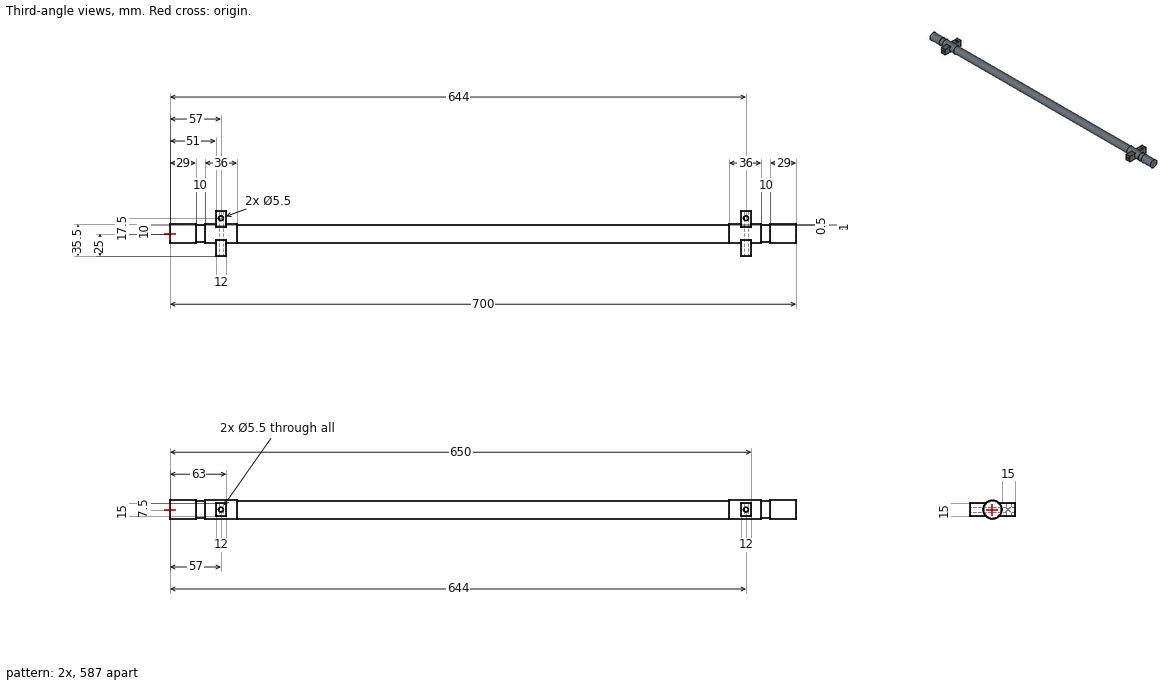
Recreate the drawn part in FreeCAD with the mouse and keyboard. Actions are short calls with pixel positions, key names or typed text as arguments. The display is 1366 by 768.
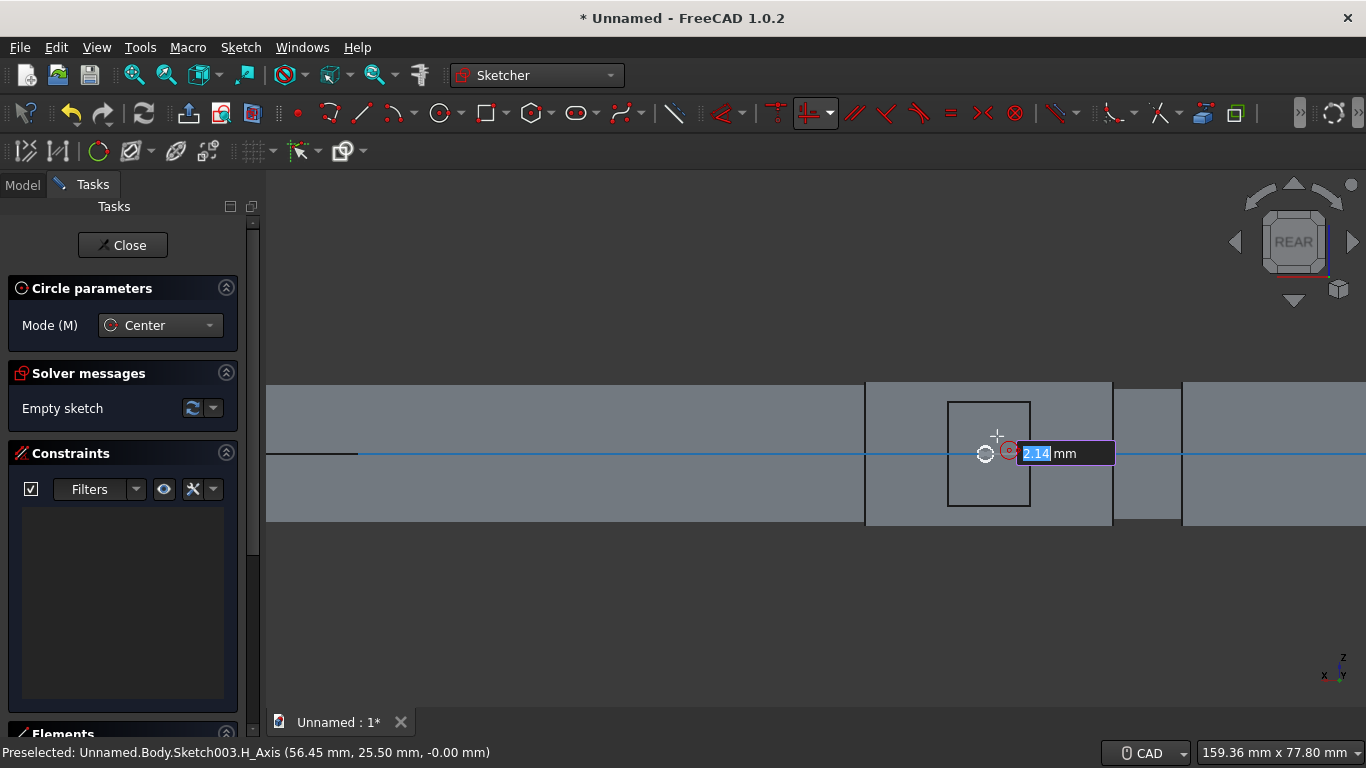
click(995, 436)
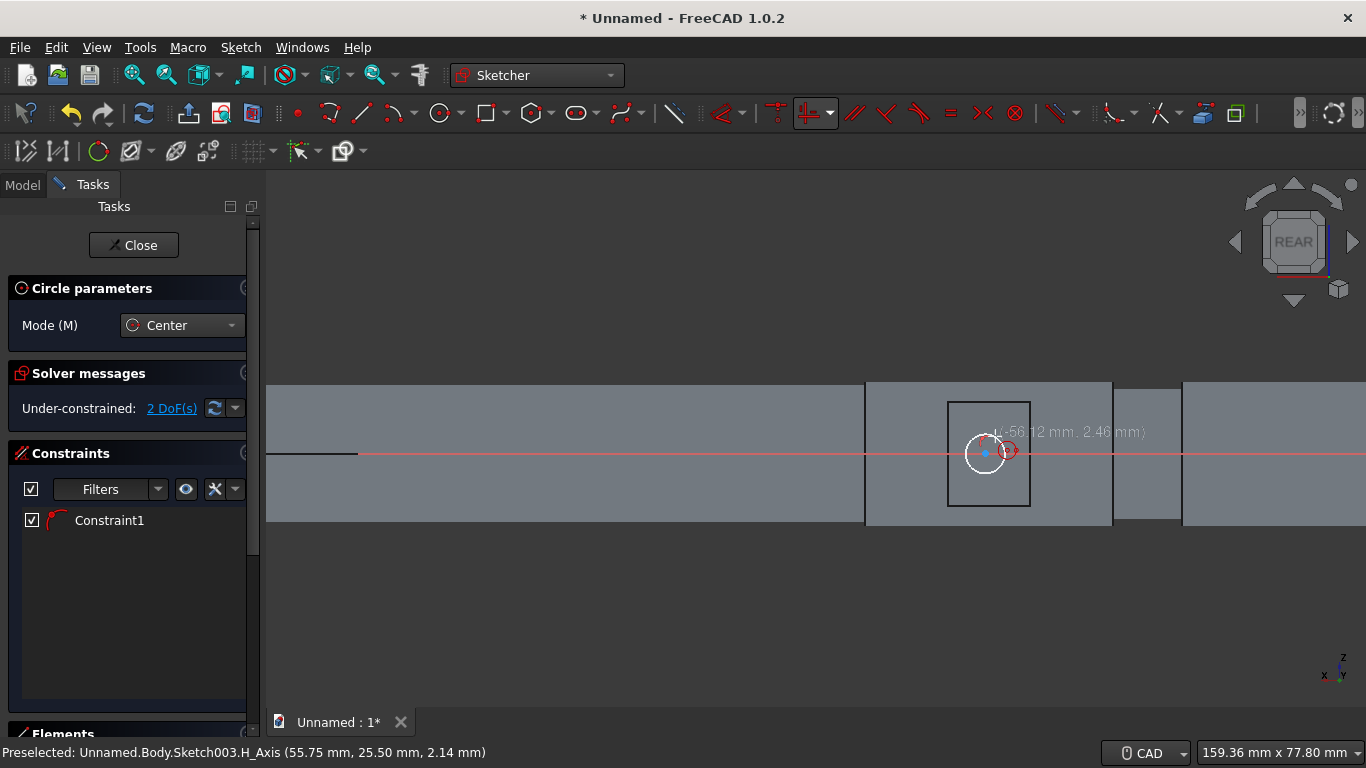
scroll(997, 436, down, 10)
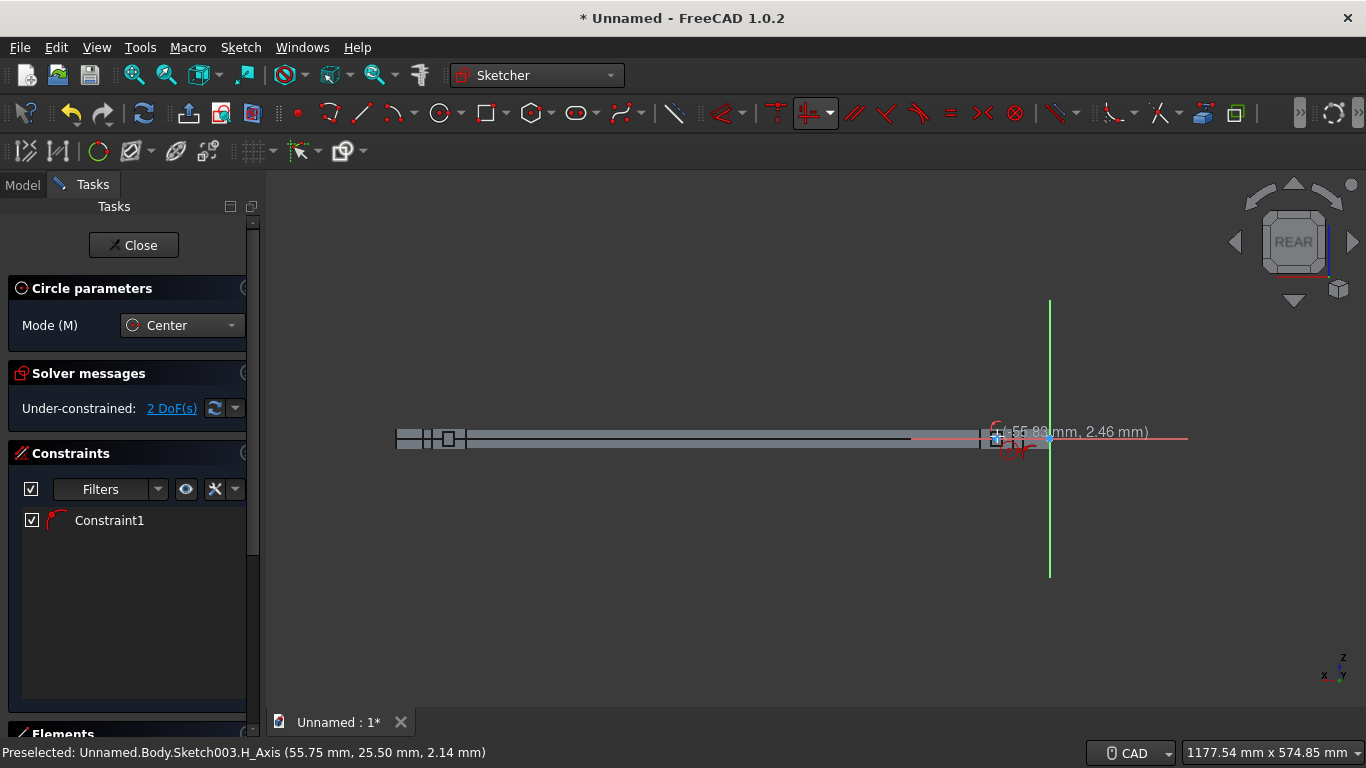
scroll(448, 439, up, 11)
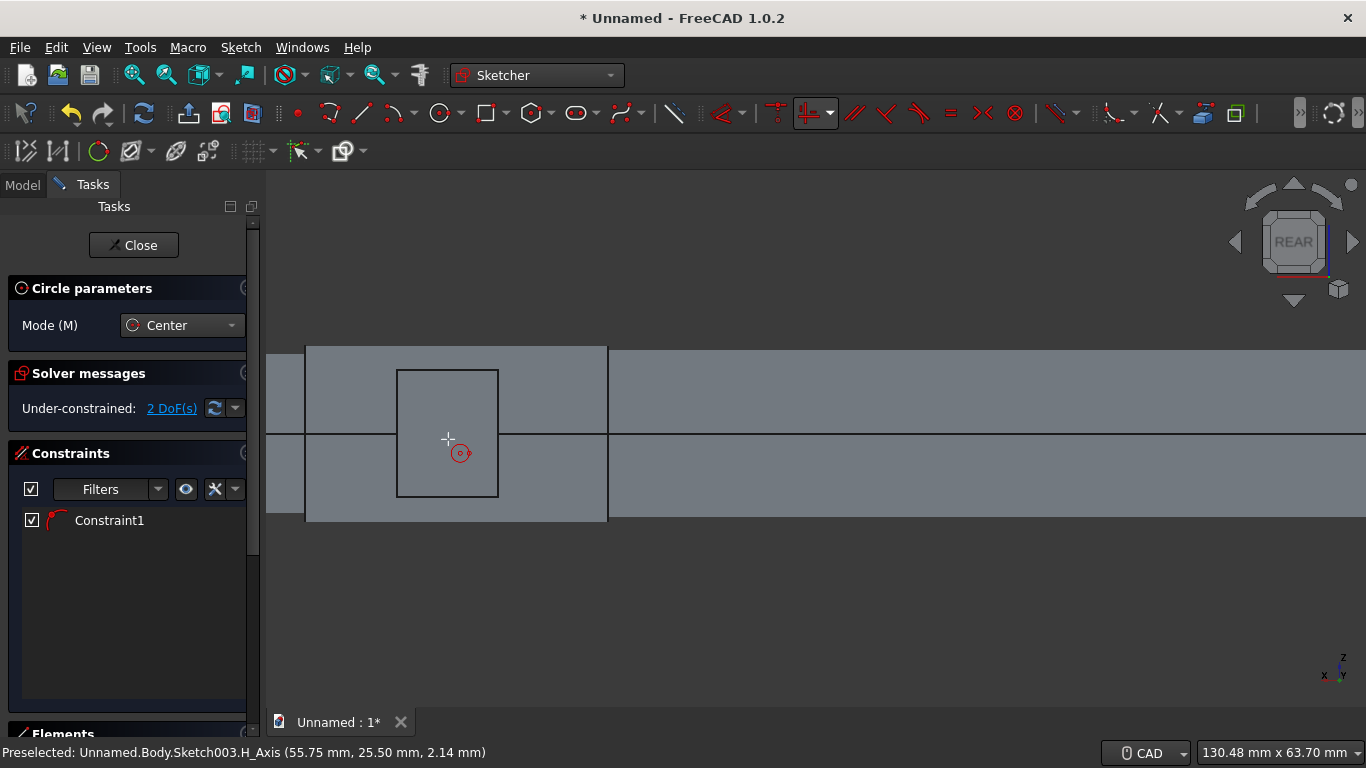
scroll(448, 439, down, 11)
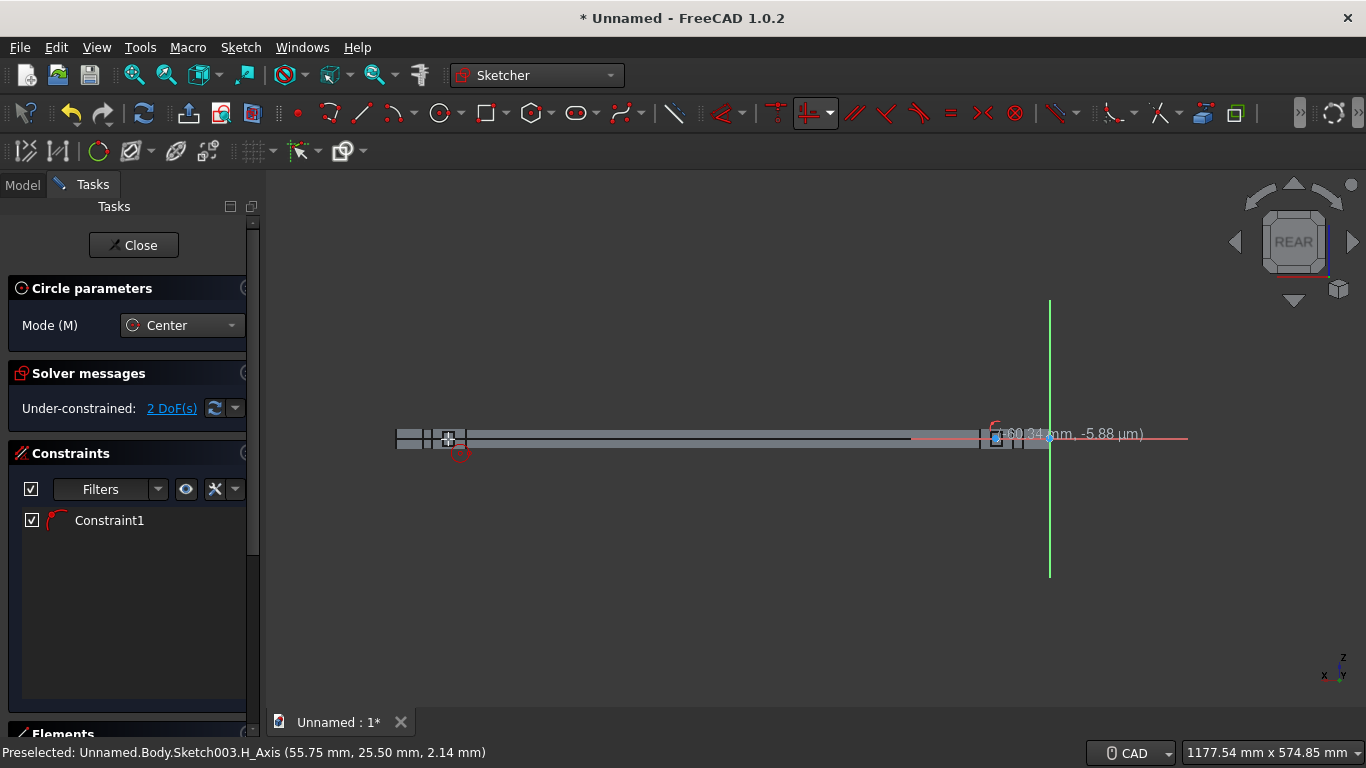
click(448, 439)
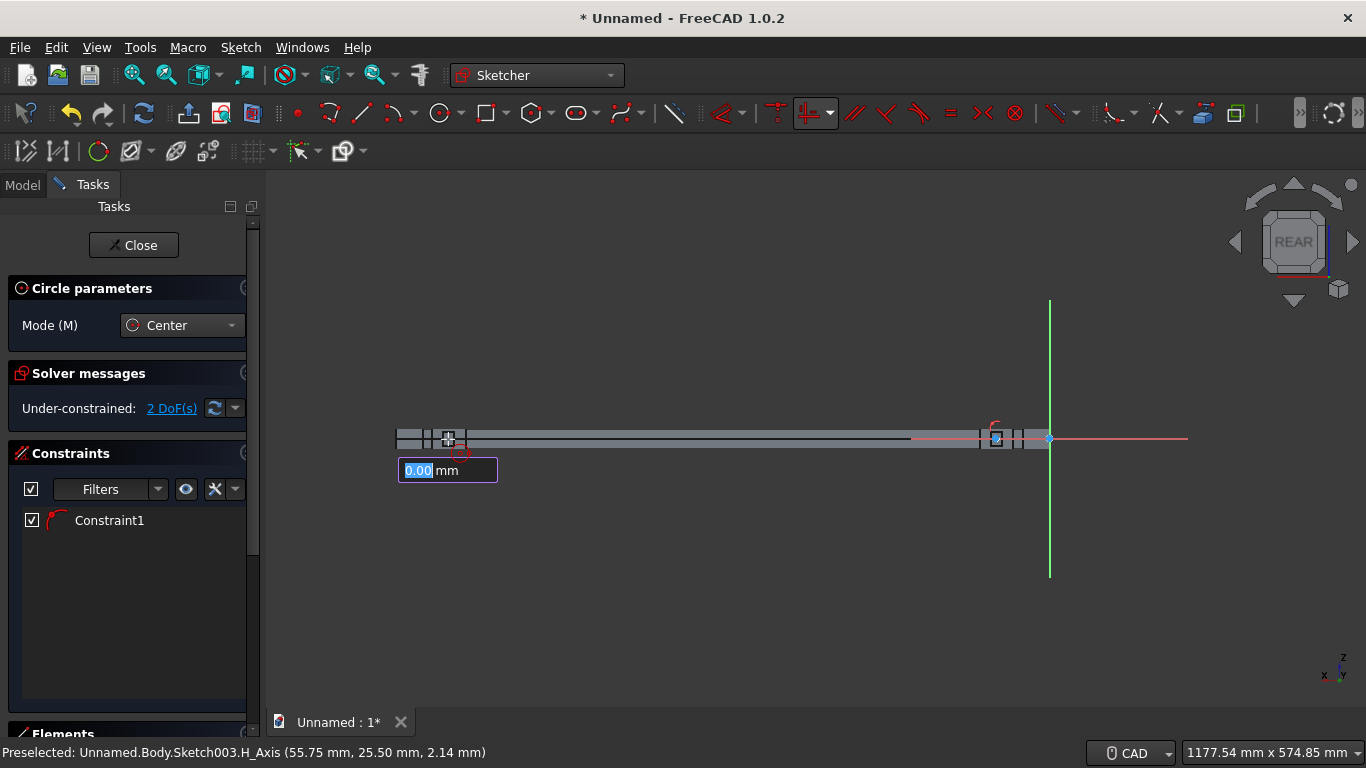
scroll(449, 436, up, 10)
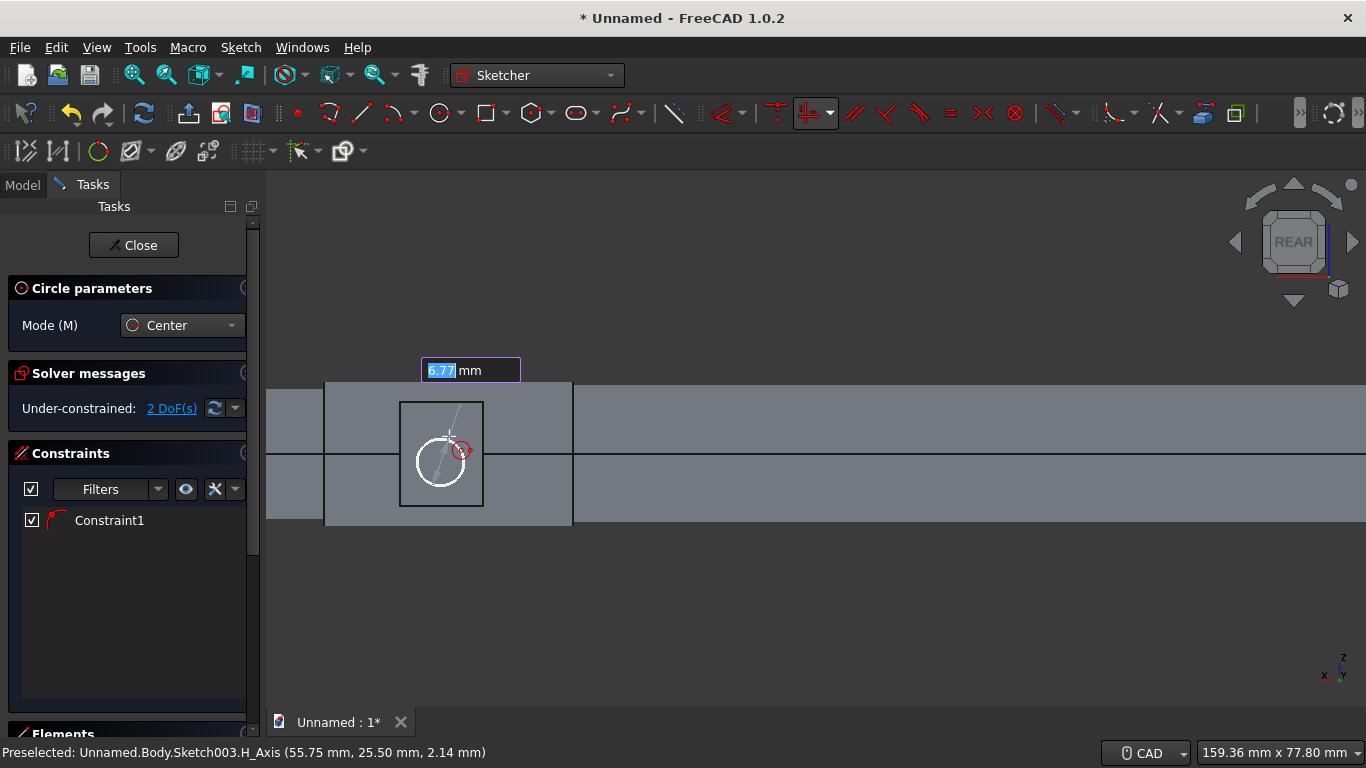
click(448, 436)
key(Escape)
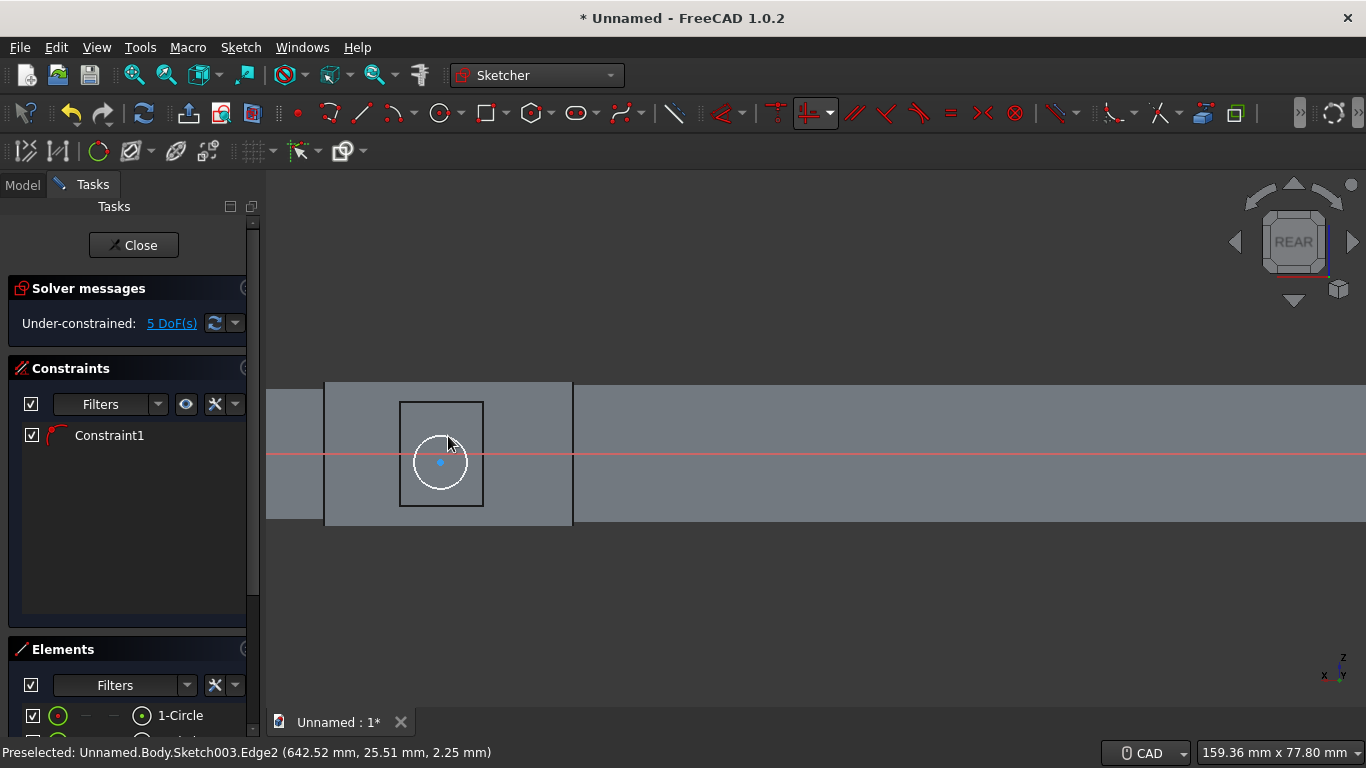
scroll(449, 436, down, 10)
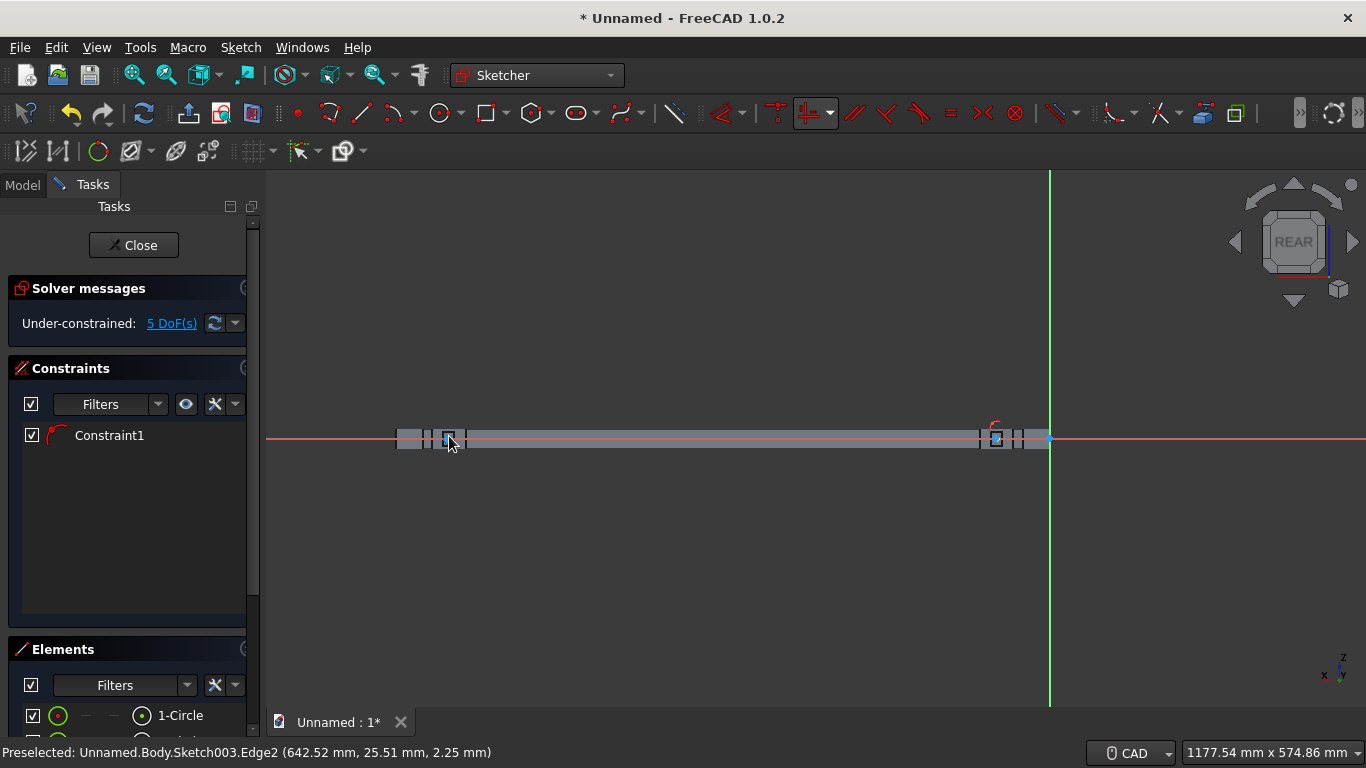
scroll(998, 437, up, 10)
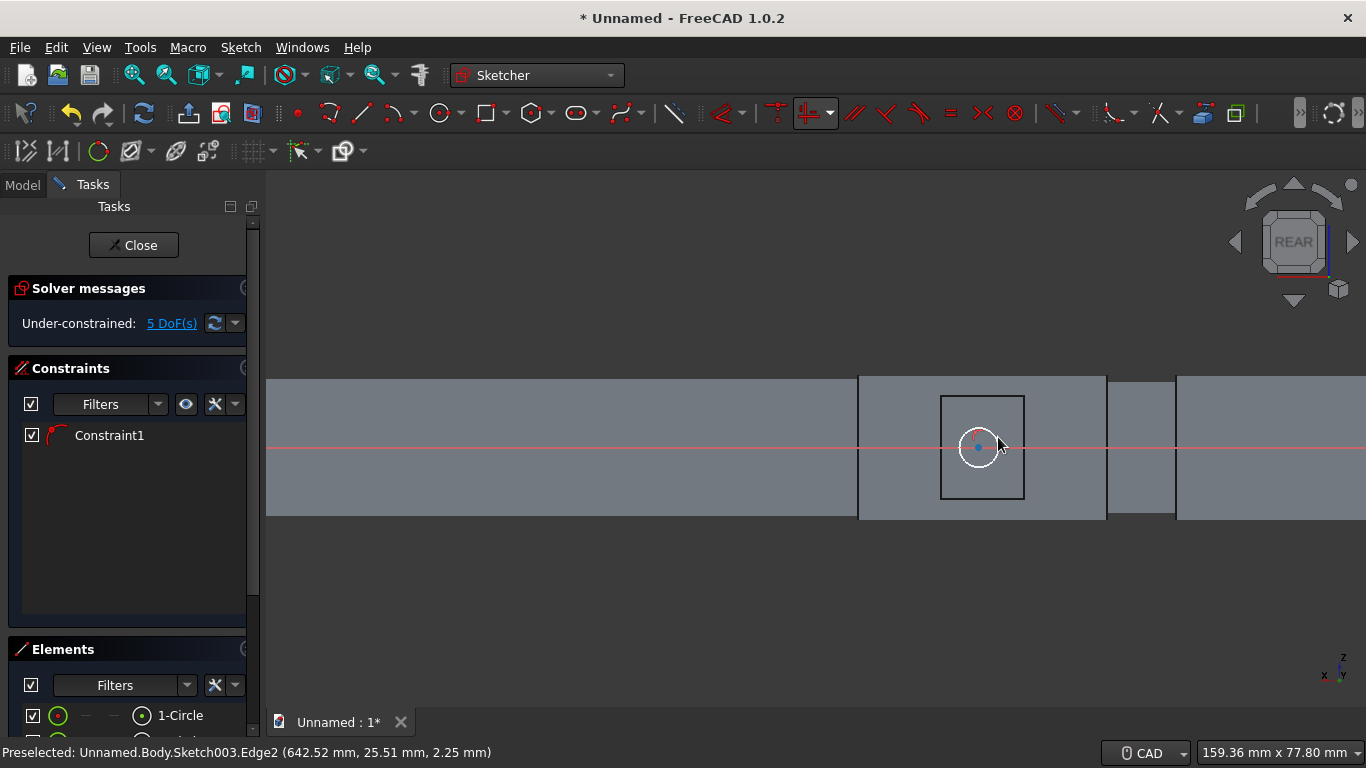
click(993, 434)